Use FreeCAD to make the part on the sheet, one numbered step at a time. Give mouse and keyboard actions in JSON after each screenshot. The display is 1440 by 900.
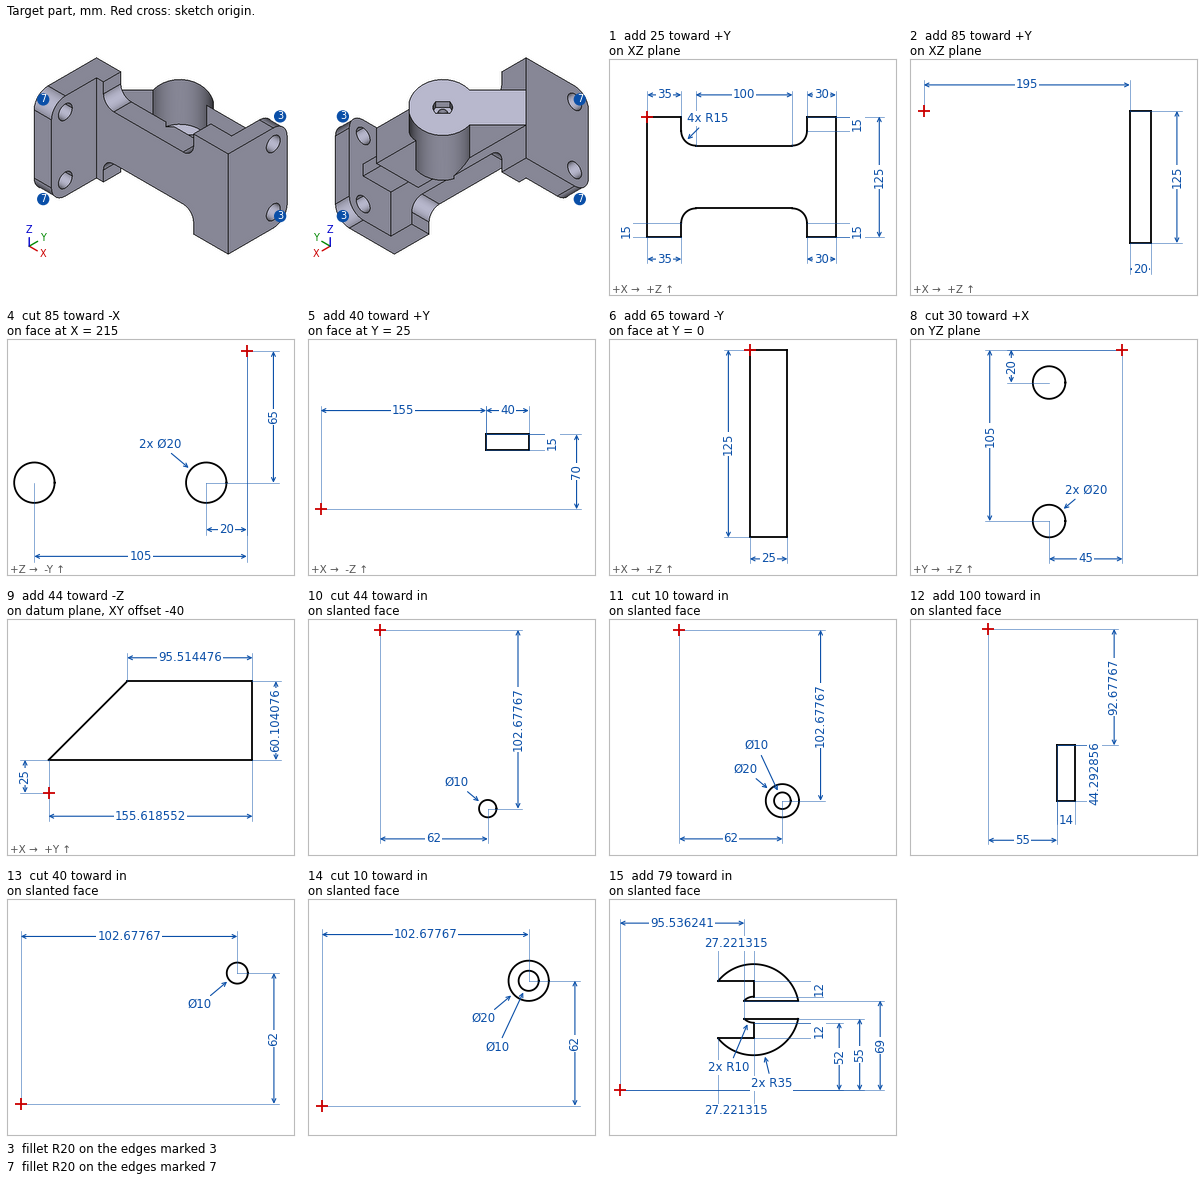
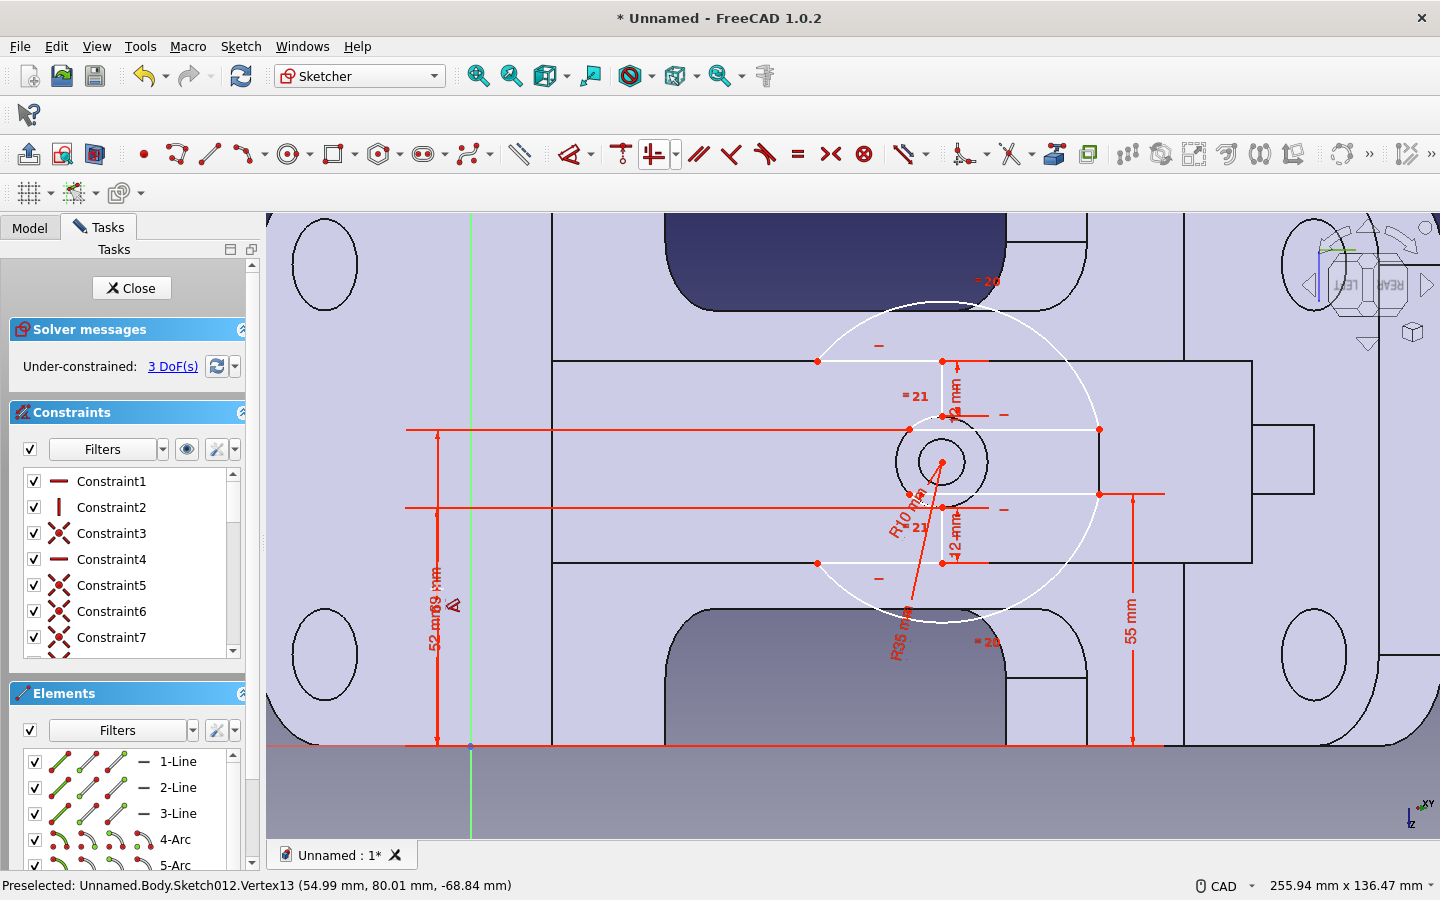
{"action": "left_click", "coordinate": [905, 563]}
{"action": "left_click", "coordinate": [908, 597]}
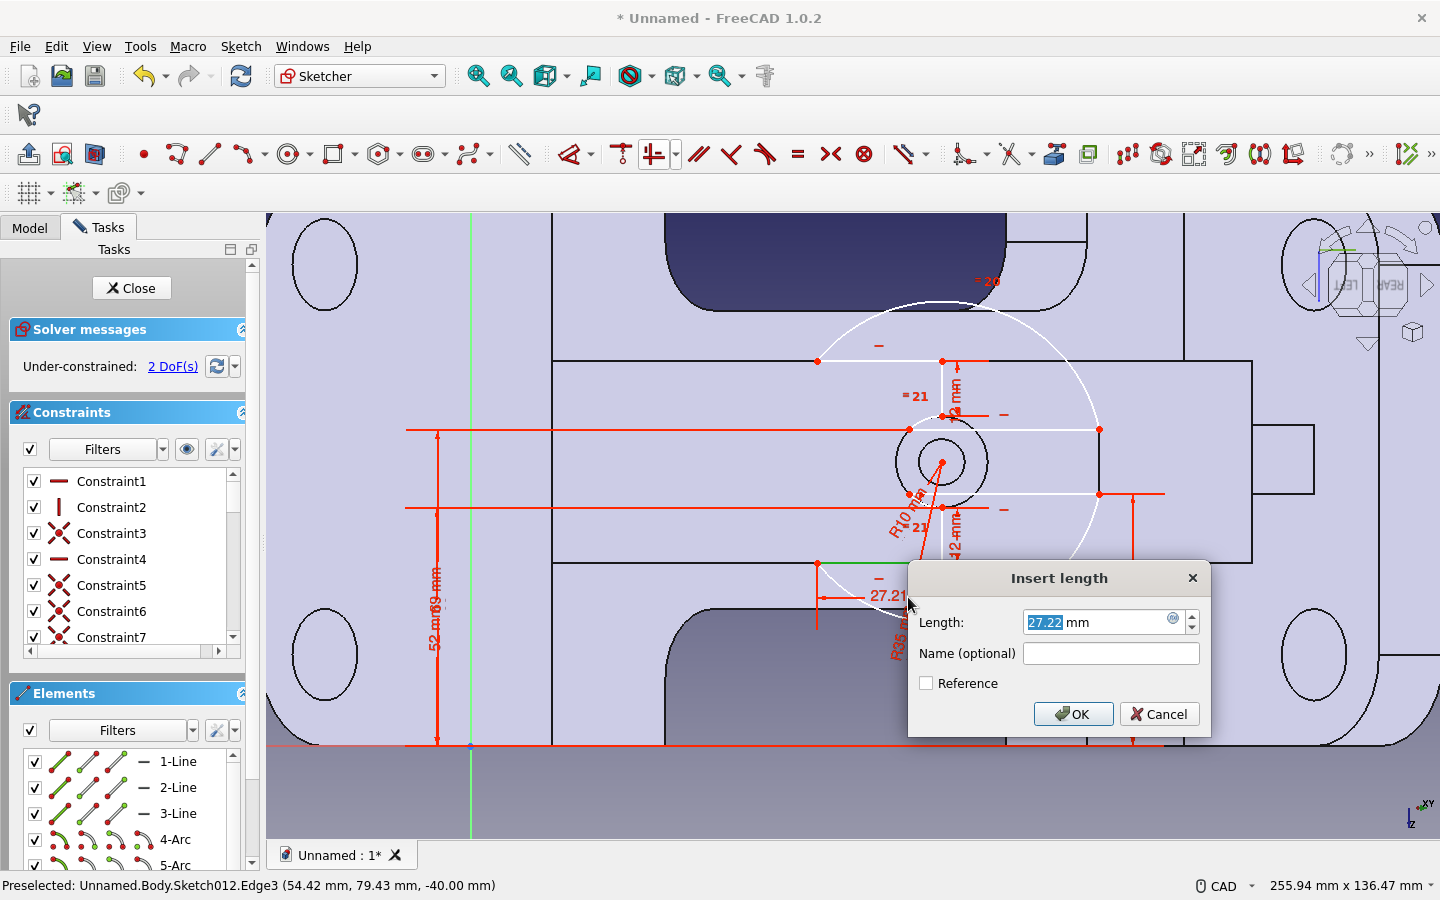
{"action": "type", "text": "27.221315"}
{"action": "key", "text": "Return"}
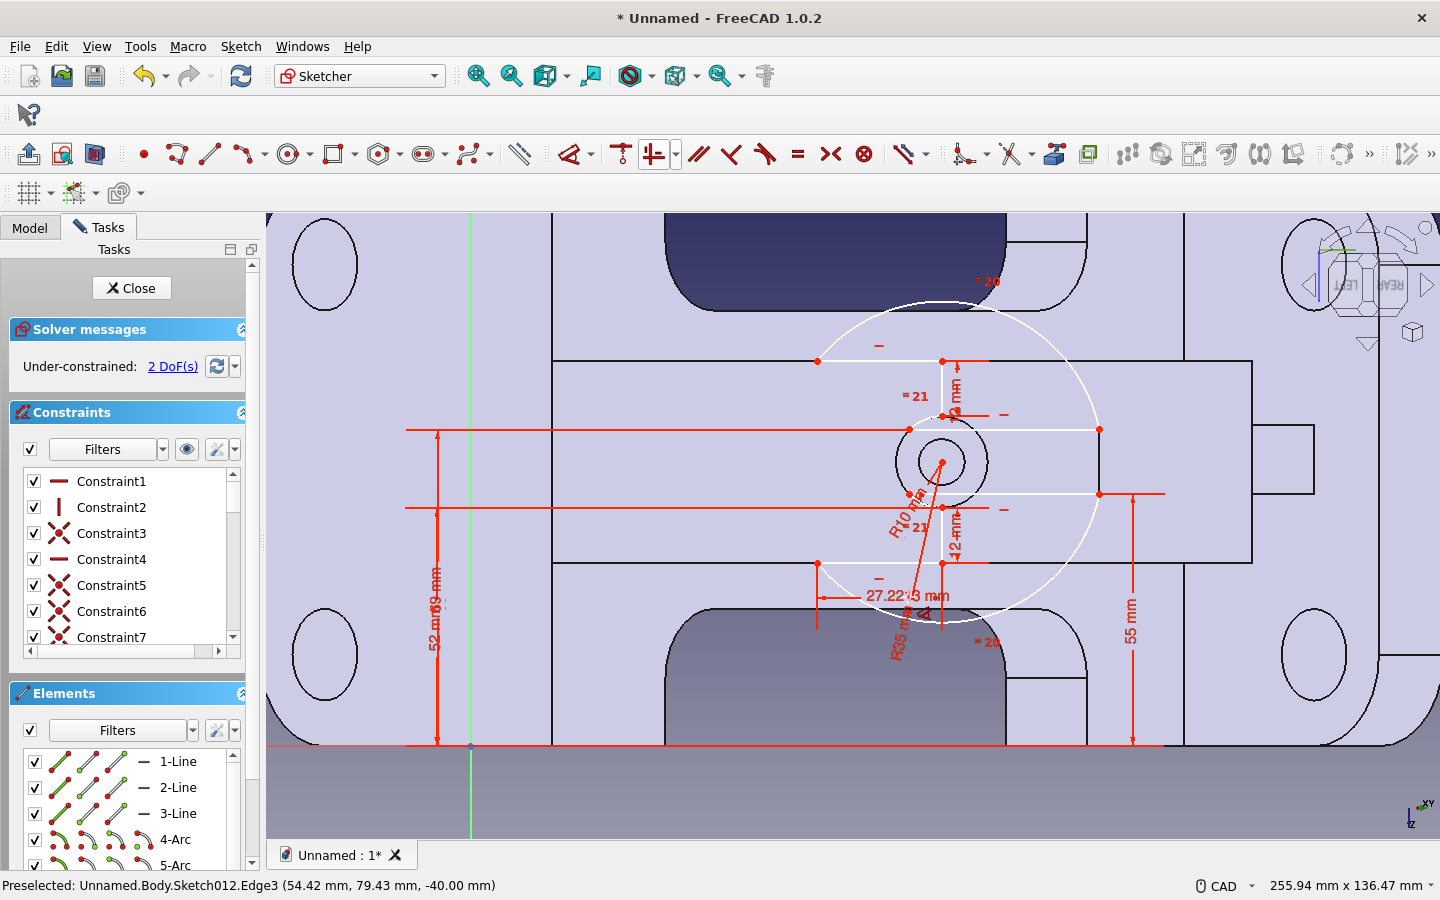
{"action": "left_click", "coordinate": [855, 361]}
{"action": "left_click", "coordinate": [909, 327]}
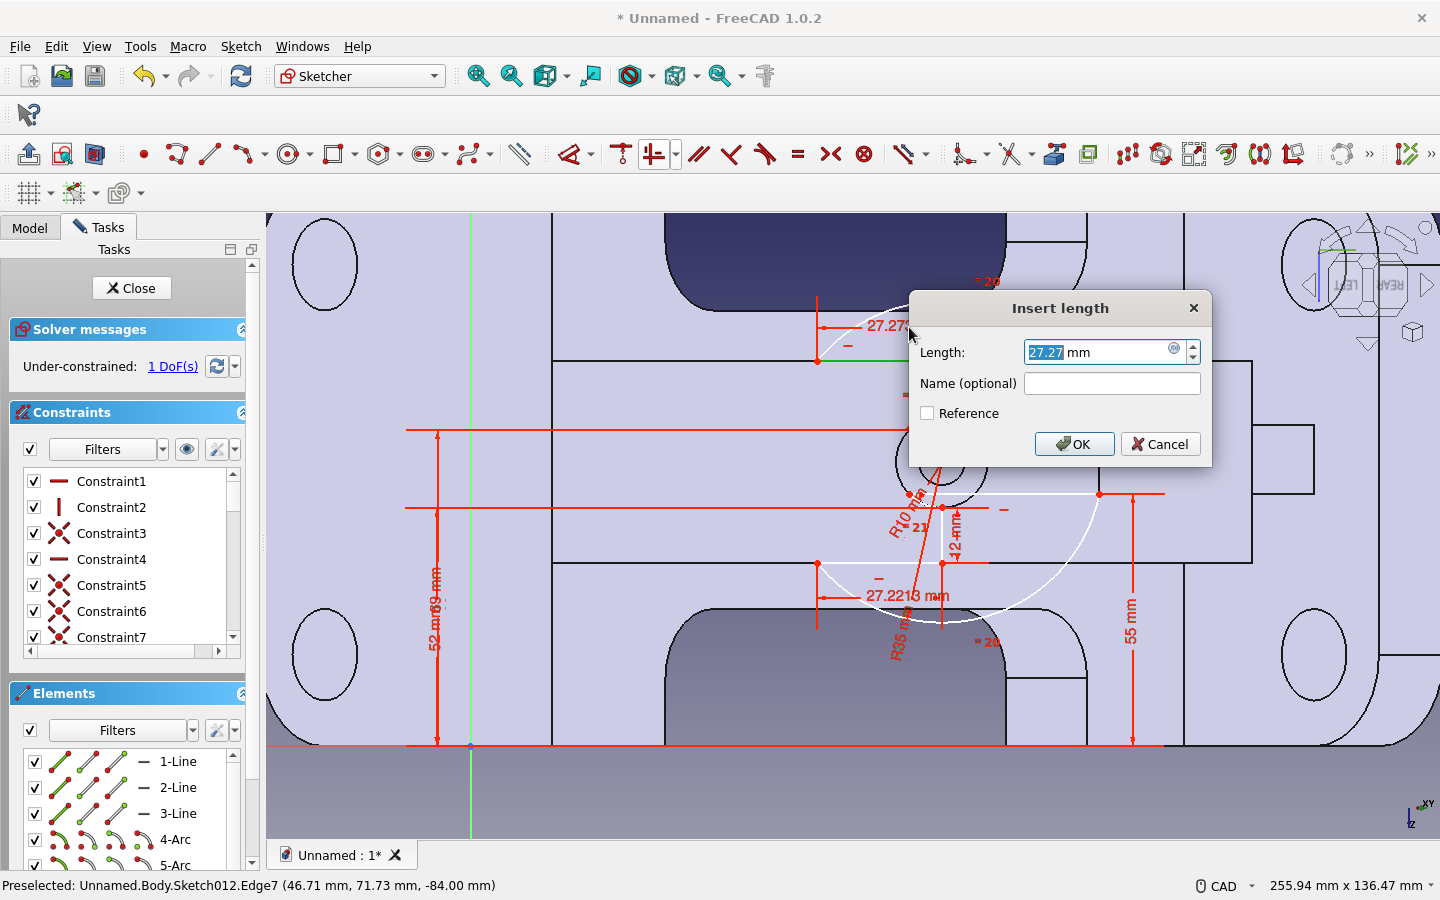
{"action": "type", "text": "27.221315"}
{"action": "key", "text": "Return"}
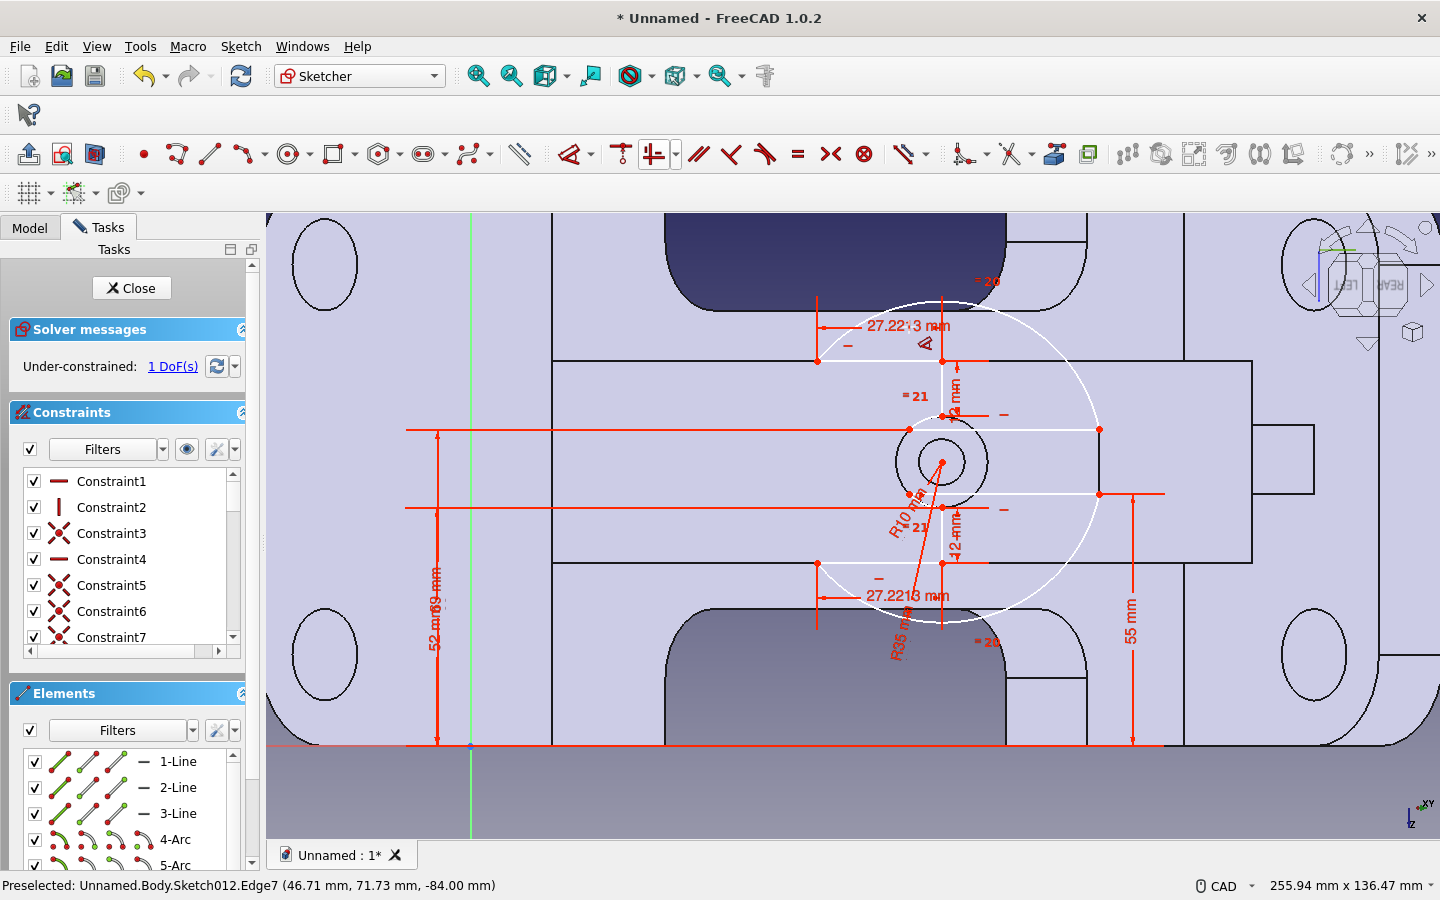
{"action": "left_click", "coordinate": [909, 494]}
{"action": "left_click", "coordinate": [690, 780]}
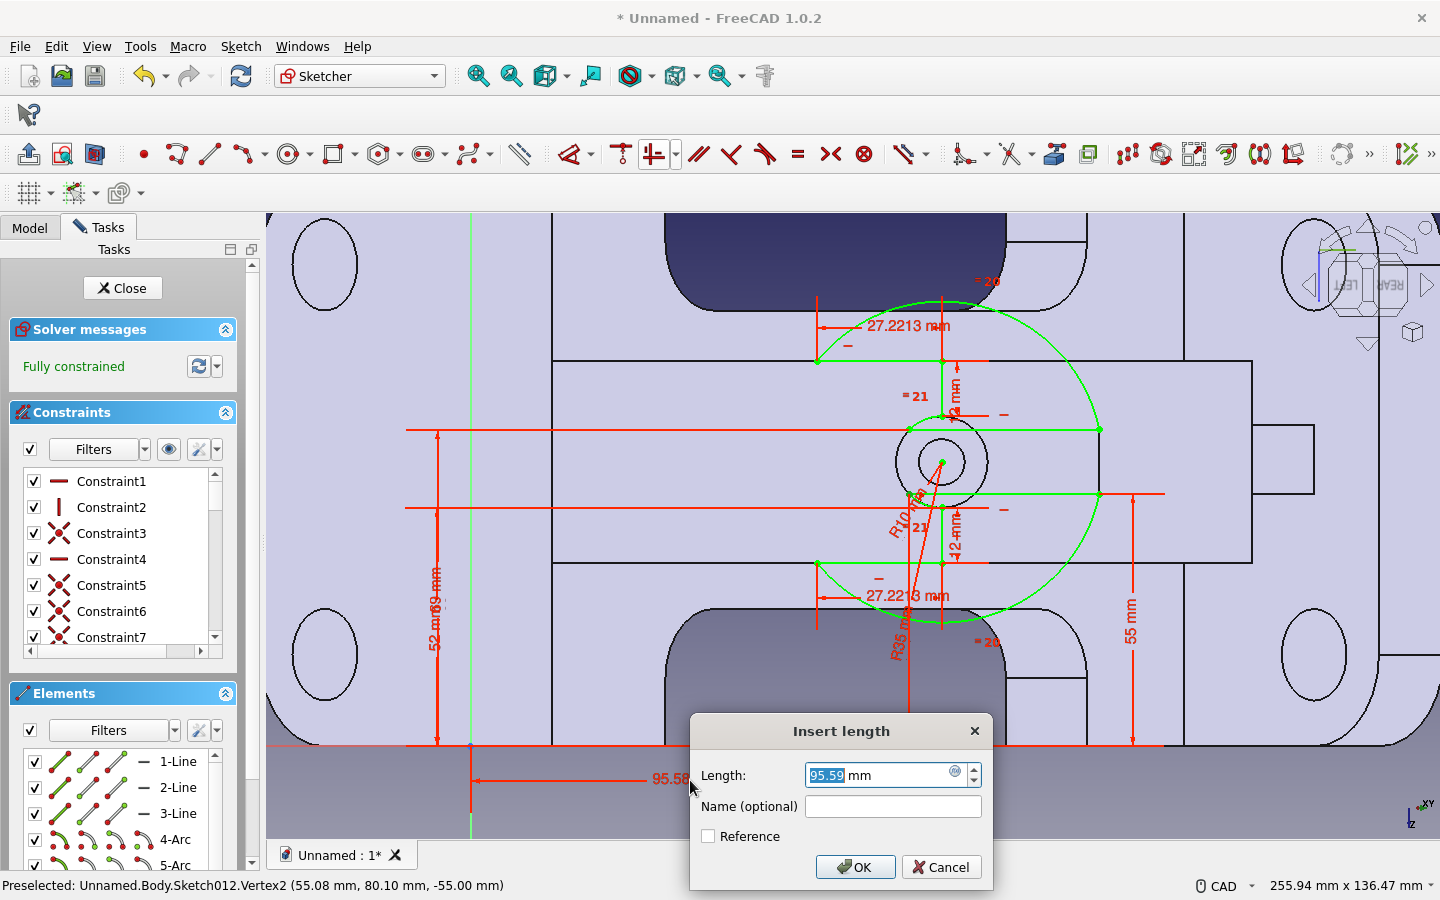
{"action": "type", "text": "95.536241"}
{"action": "key", "text": "Return"}
{"action": "key", "text": "Escape"}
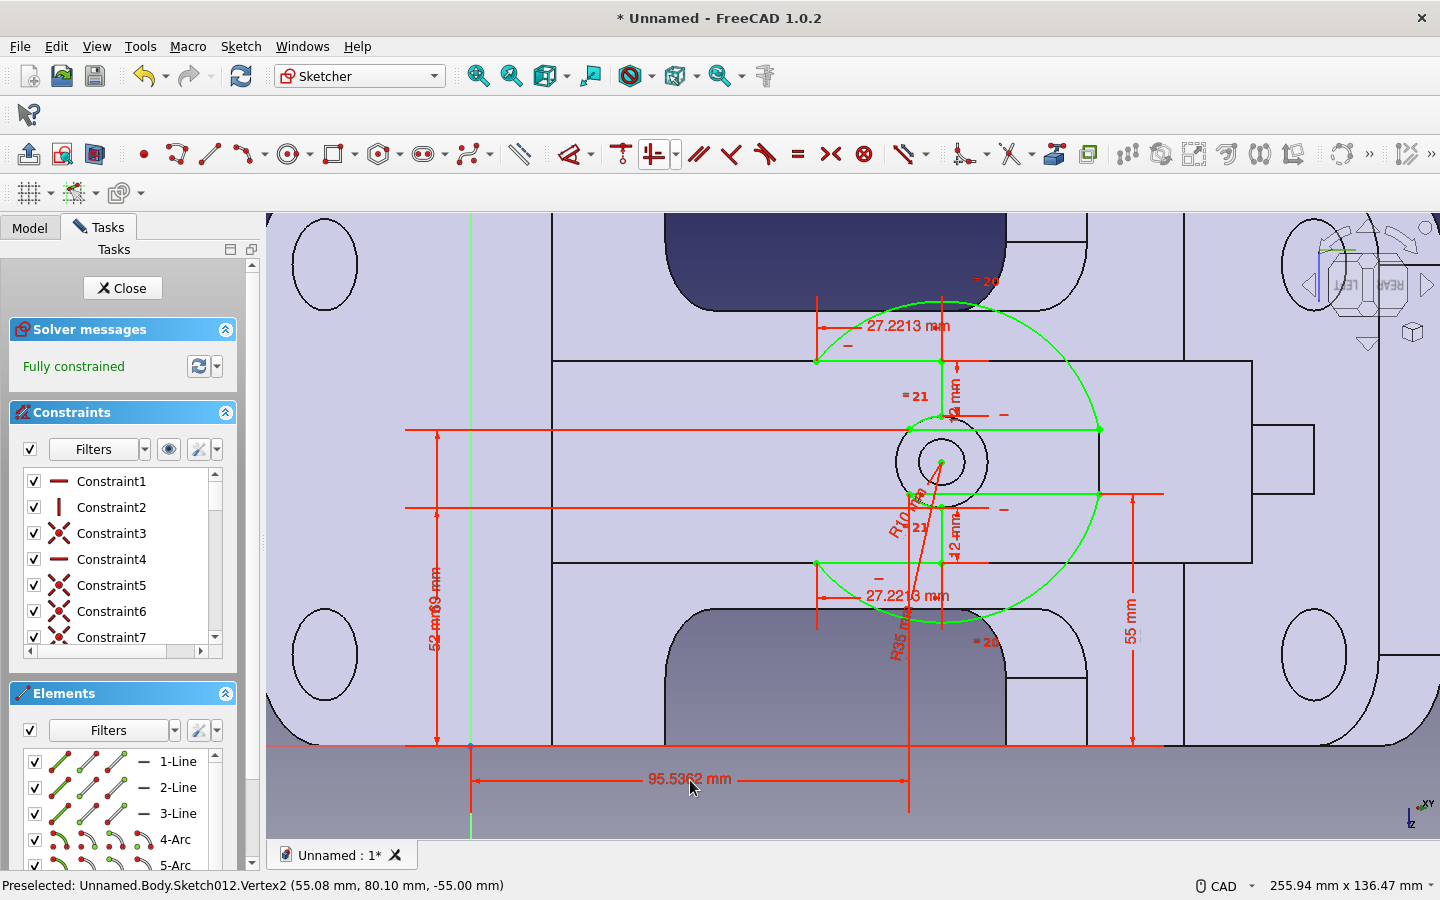
{"action": "left_click", "coordinate": [123, 288]}